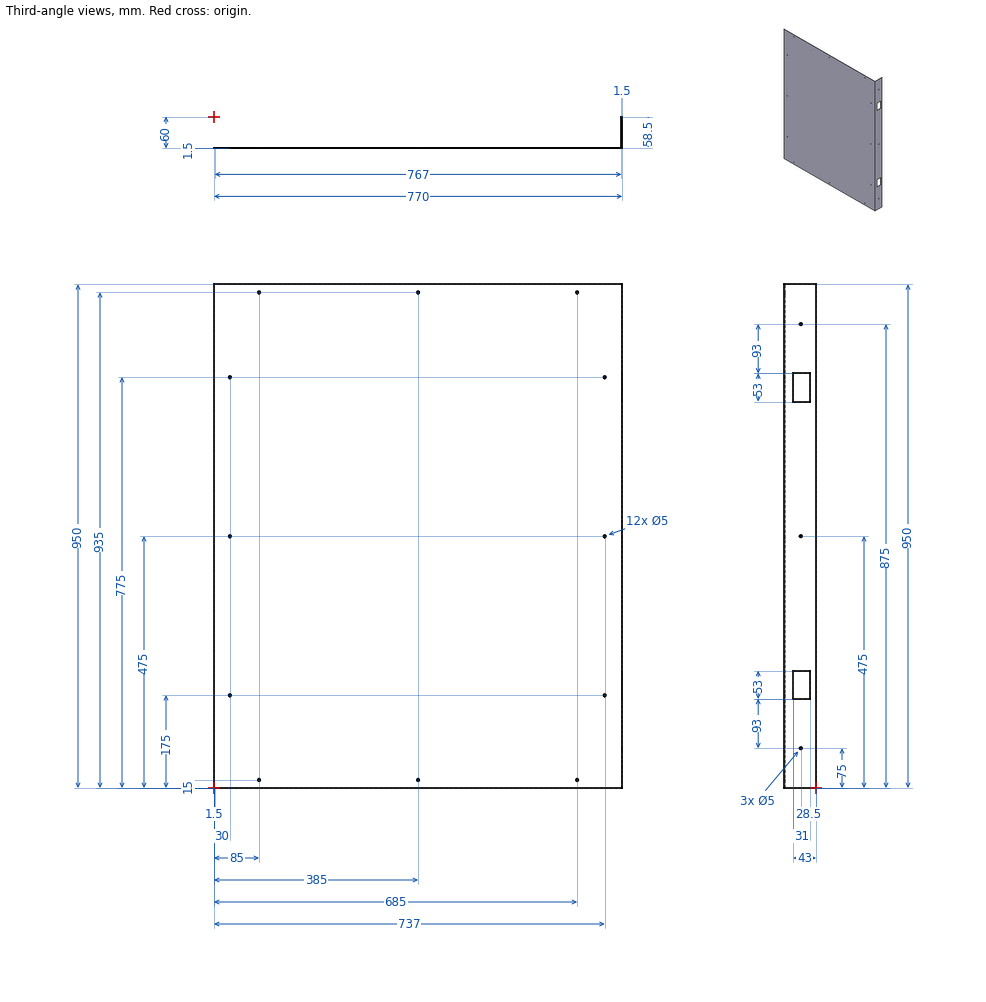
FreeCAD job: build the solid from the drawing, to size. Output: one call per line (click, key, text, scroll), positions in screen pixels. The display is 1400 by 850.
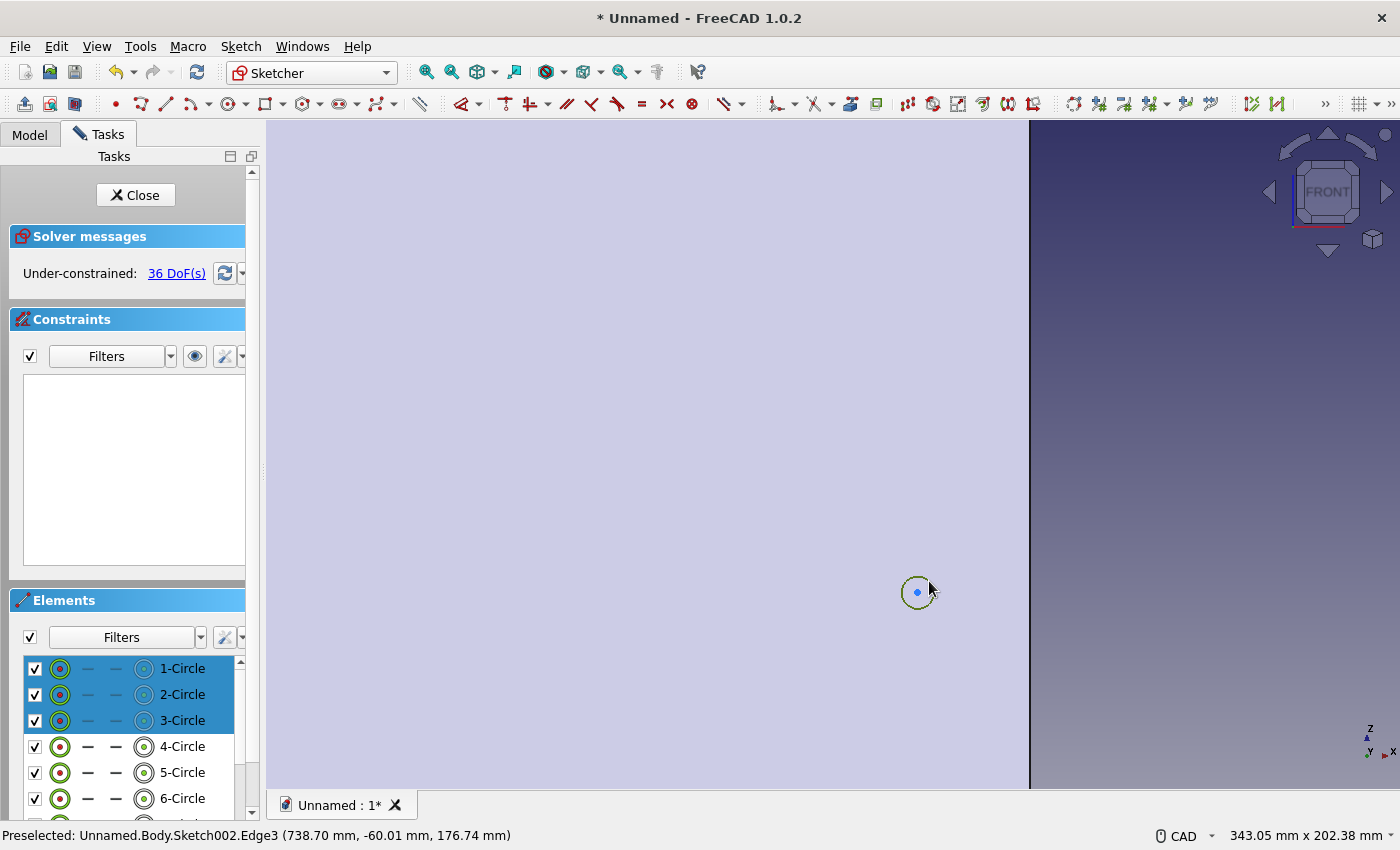
scroll(930, 586, down, 10)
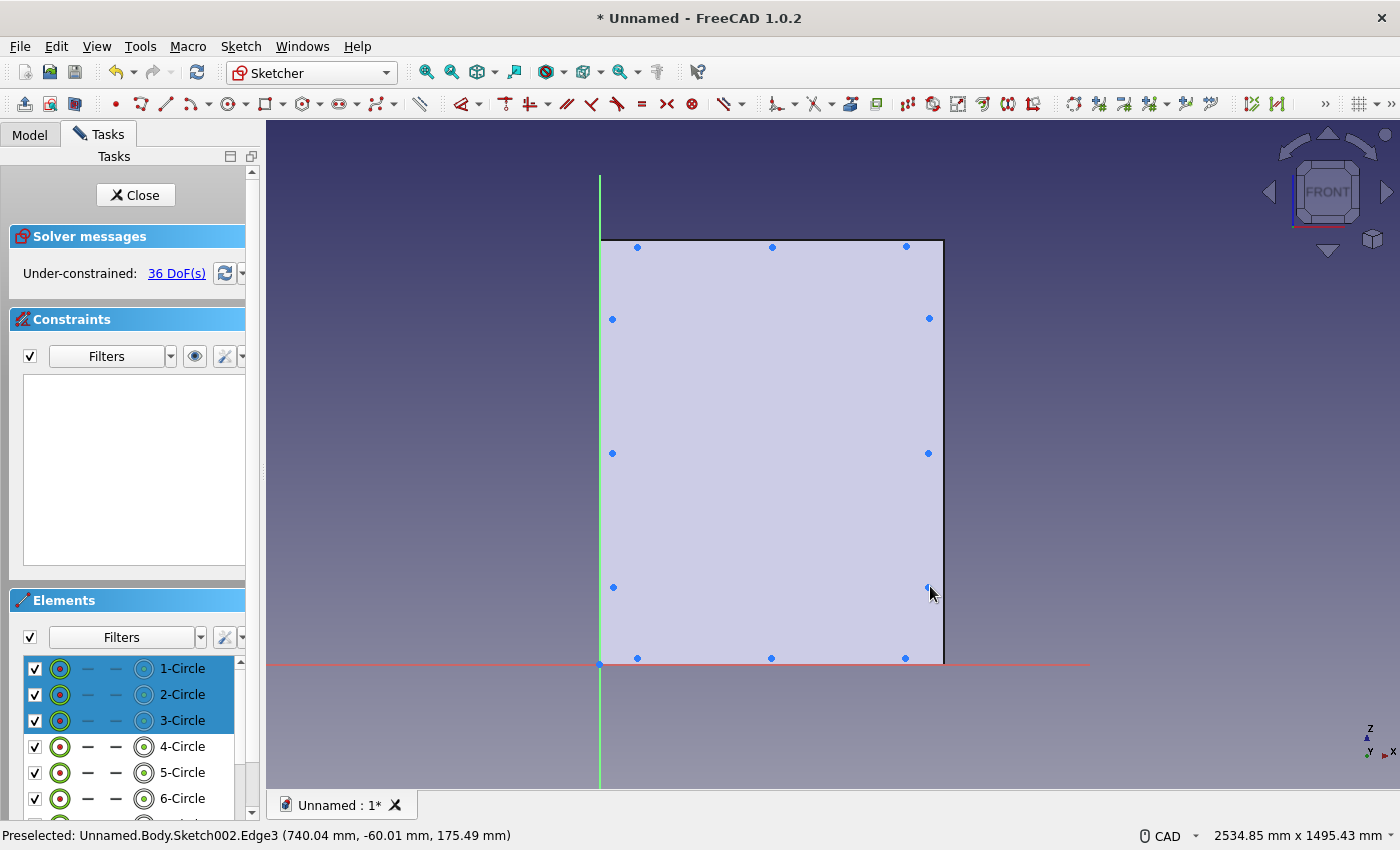
scroll(614, 318, up, 10)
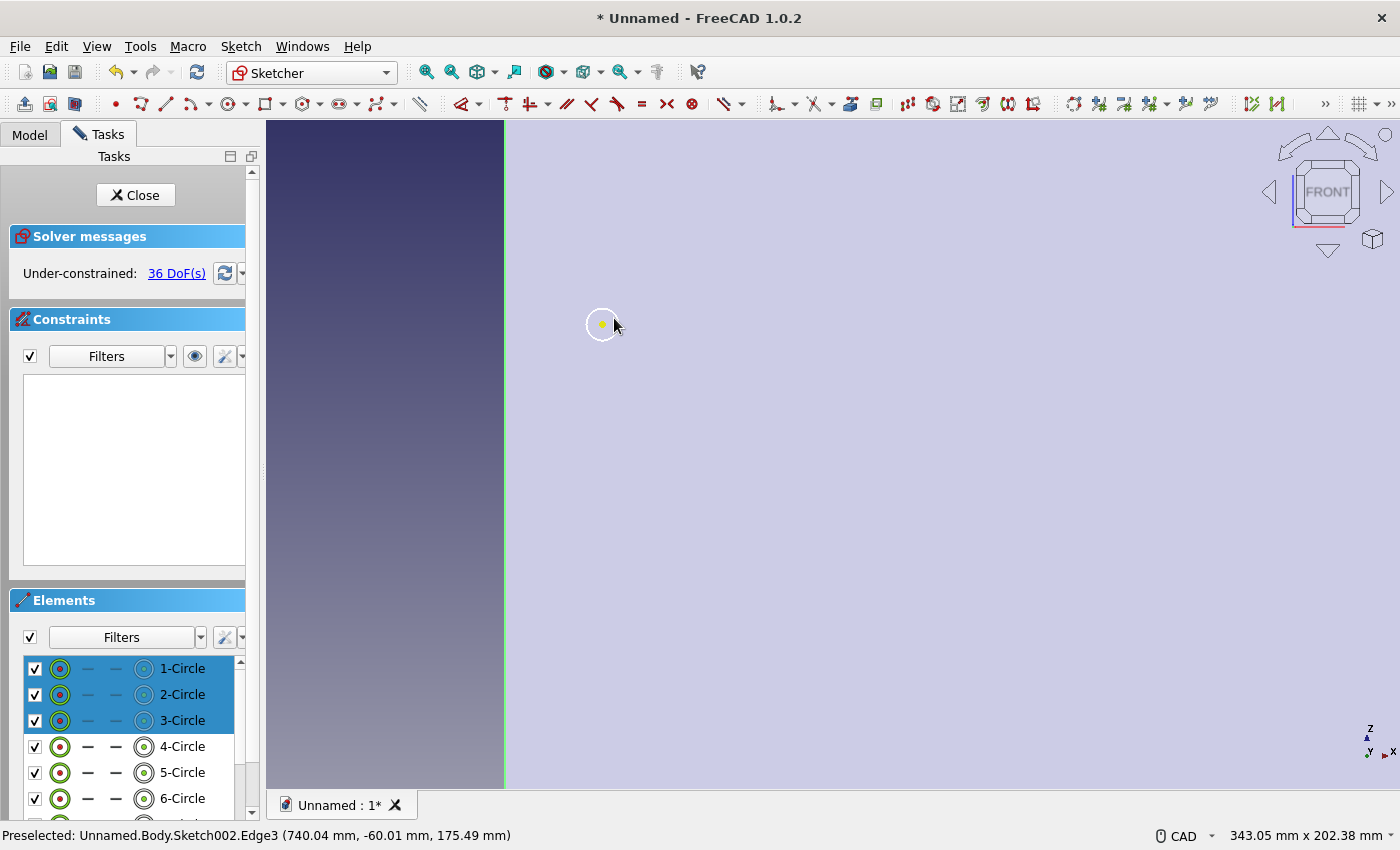
click(614, 313)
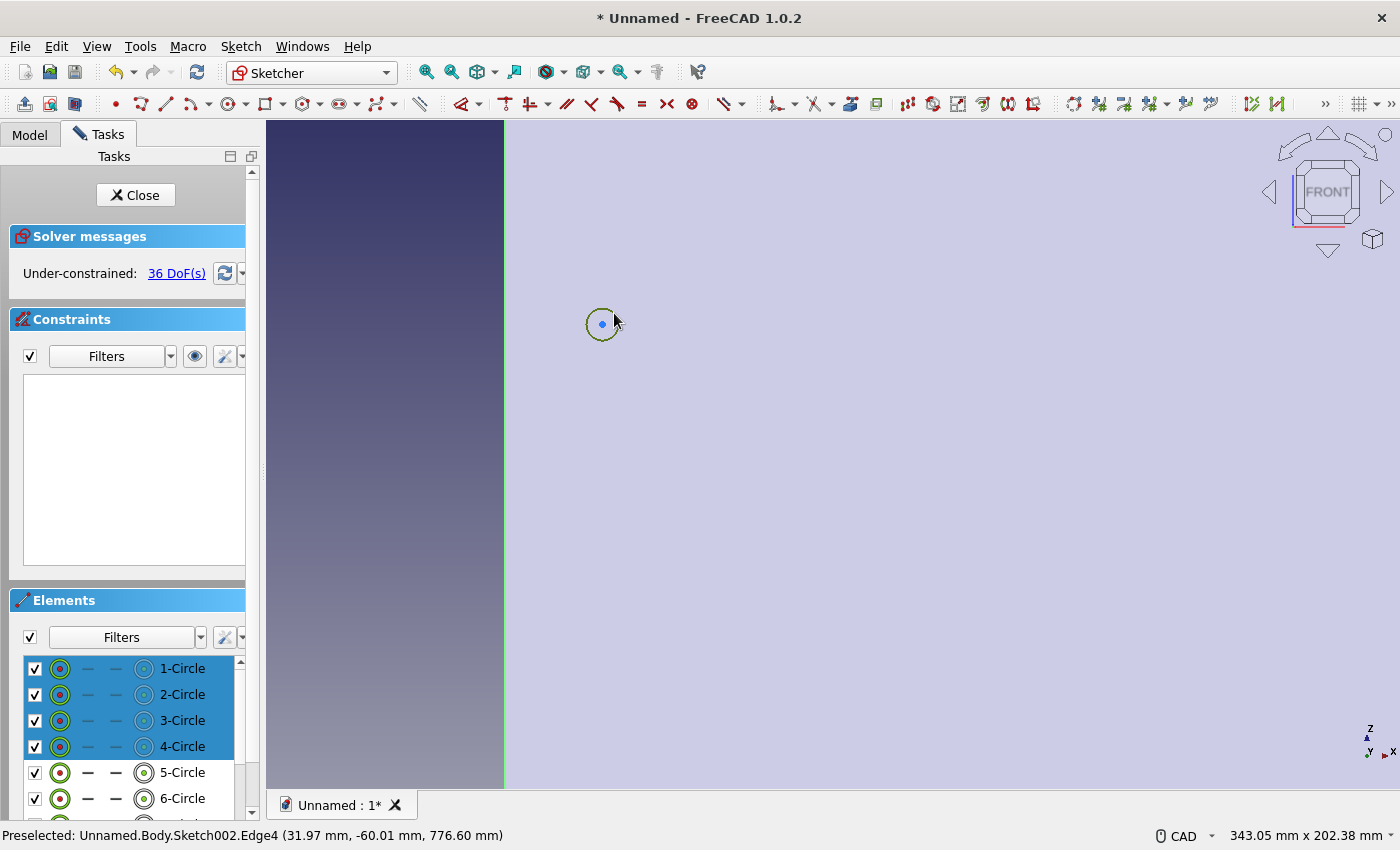
scroll(614, 318, down, 10)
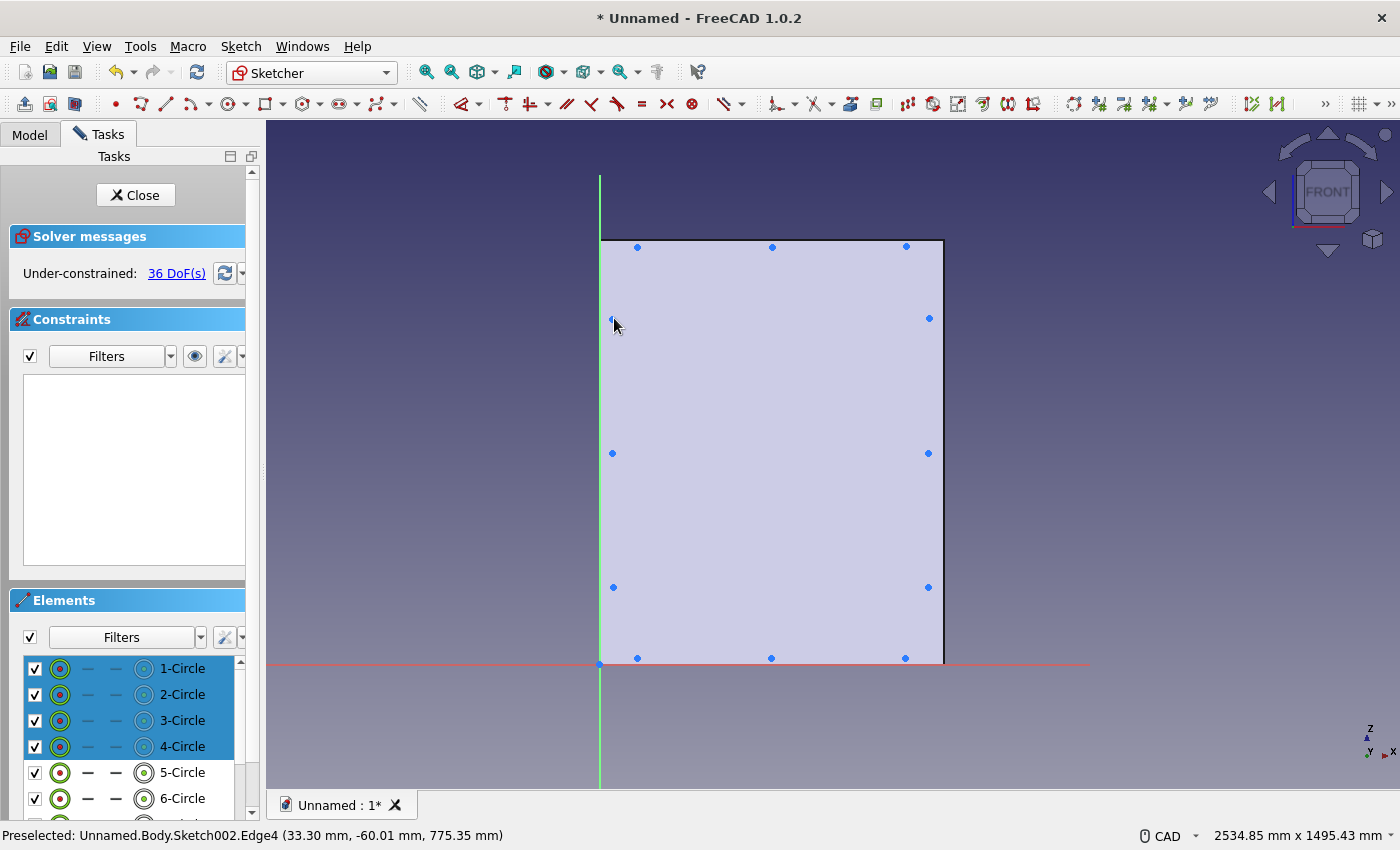
scroll(614, 452, up, 10)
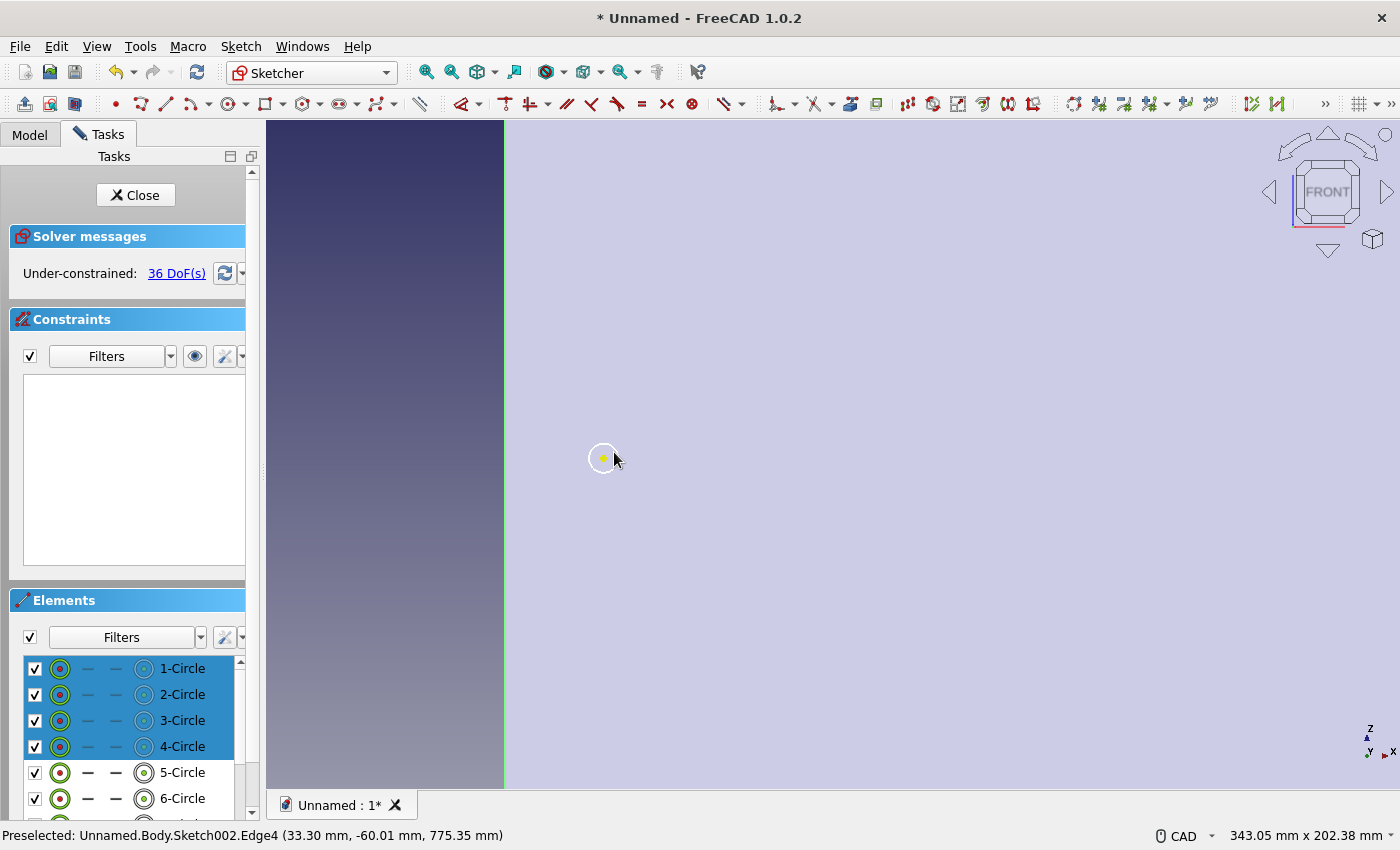
click(614, 448)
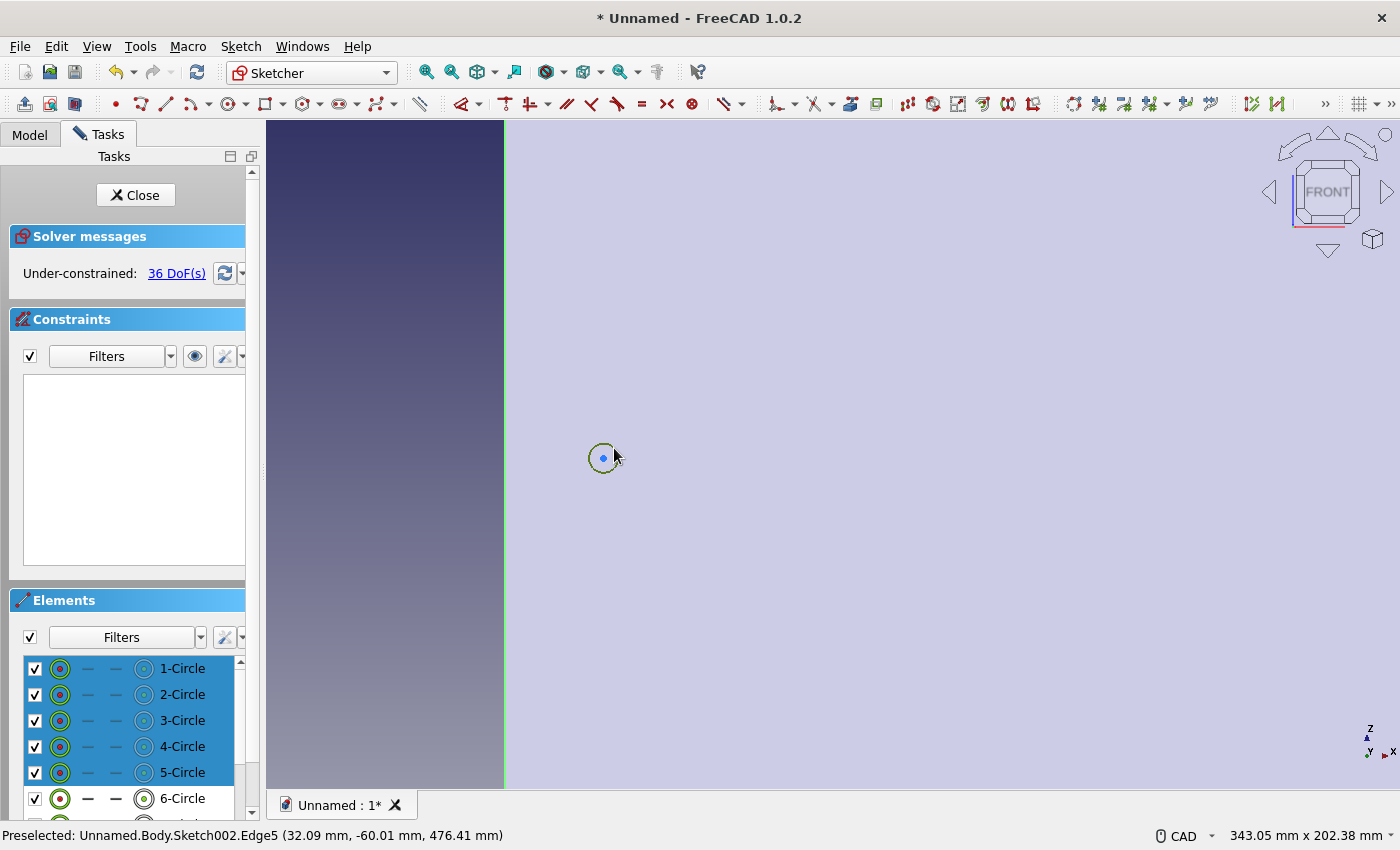
scroll(614, 452, down, 10)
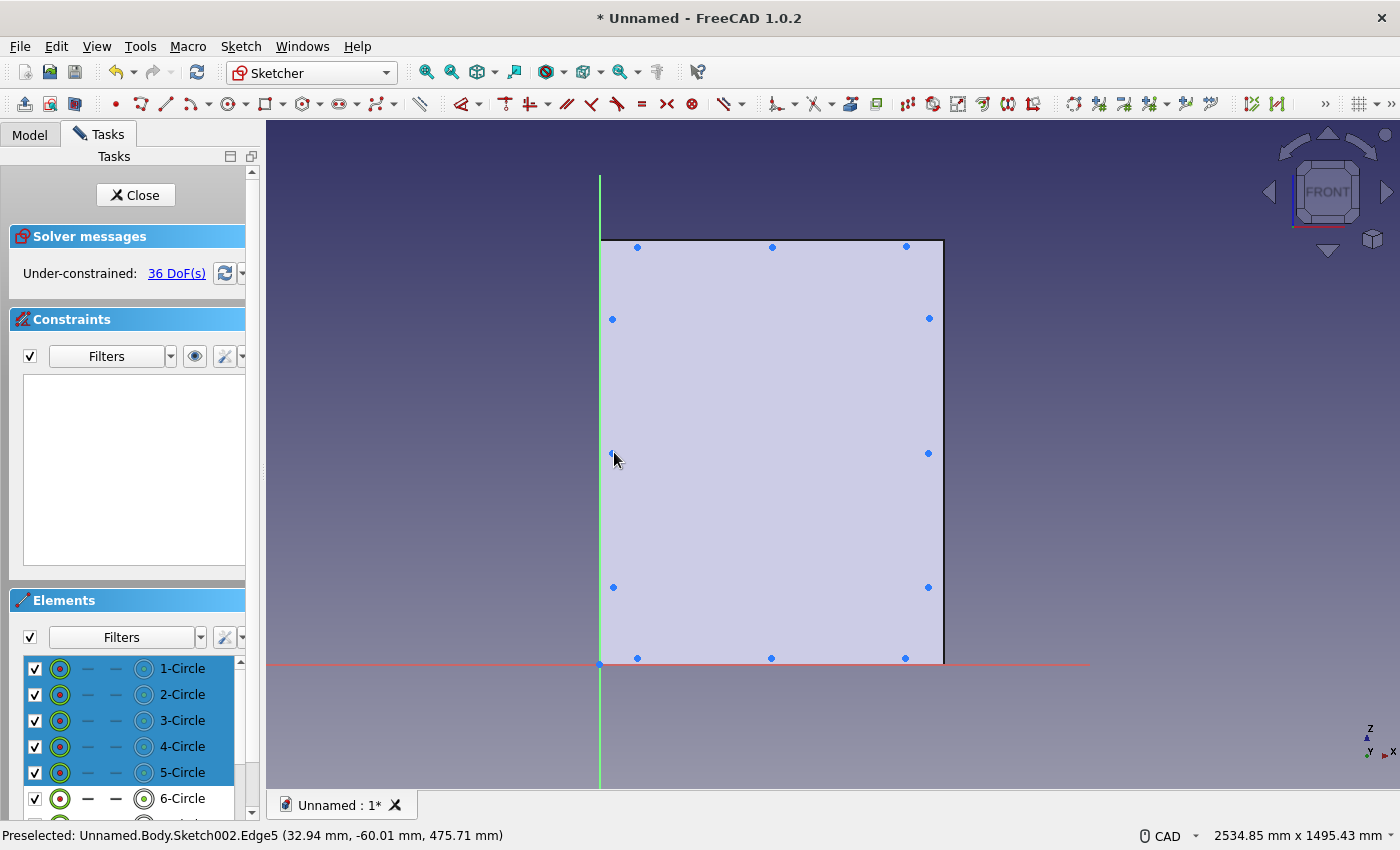
scroll(614, 586, up, 11)